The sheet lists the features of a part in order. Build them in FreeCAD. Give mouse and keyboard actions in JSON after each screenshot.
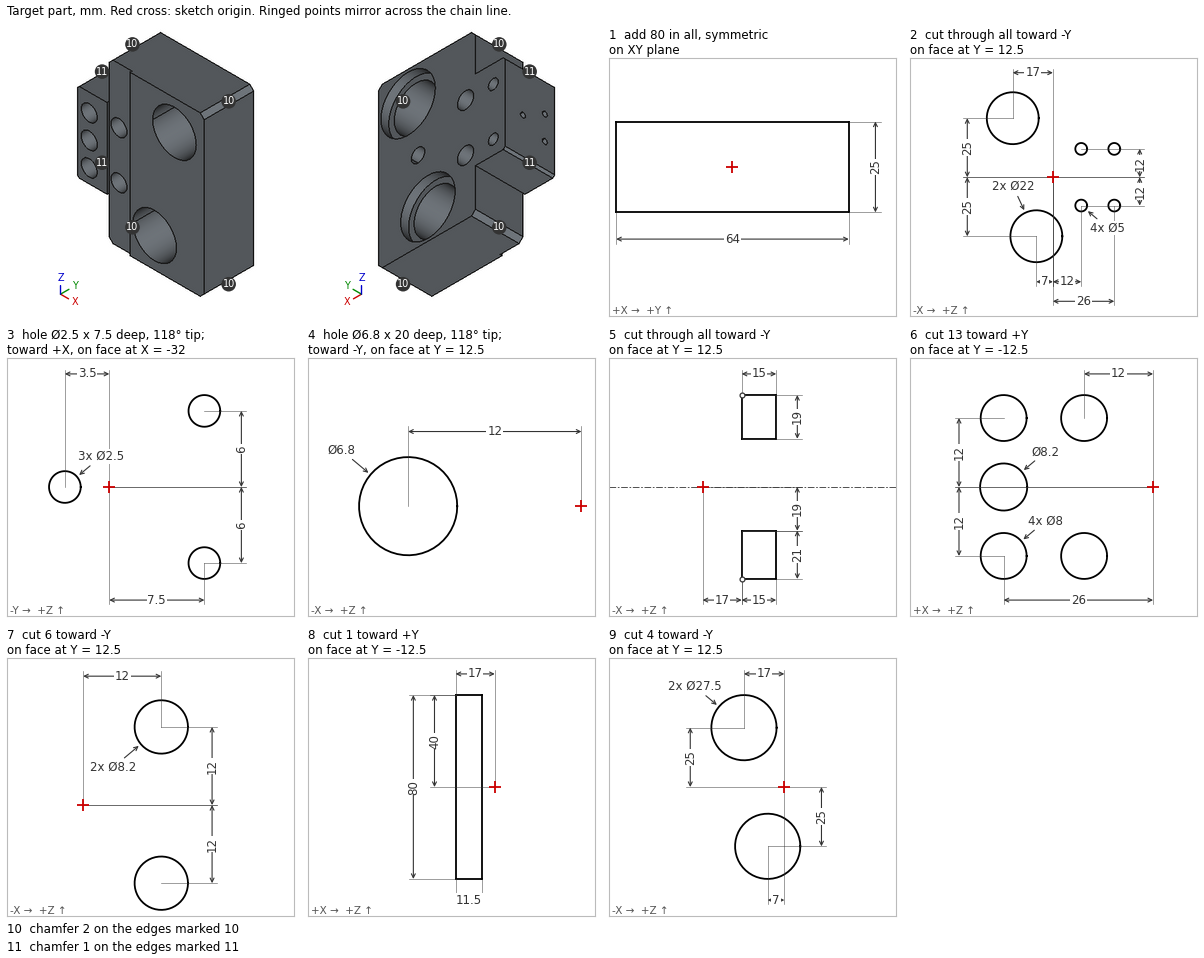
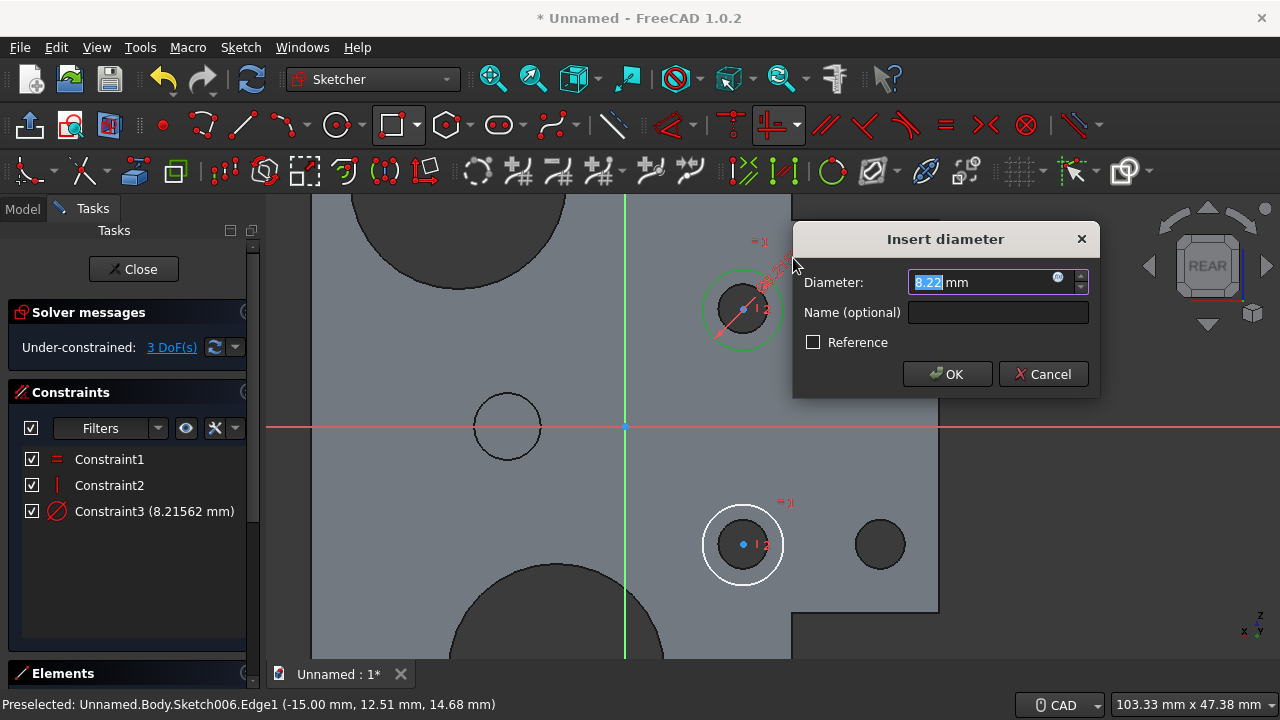
{"action": "type", "text": "8.2"}
{"action": "key", "text": "Return"}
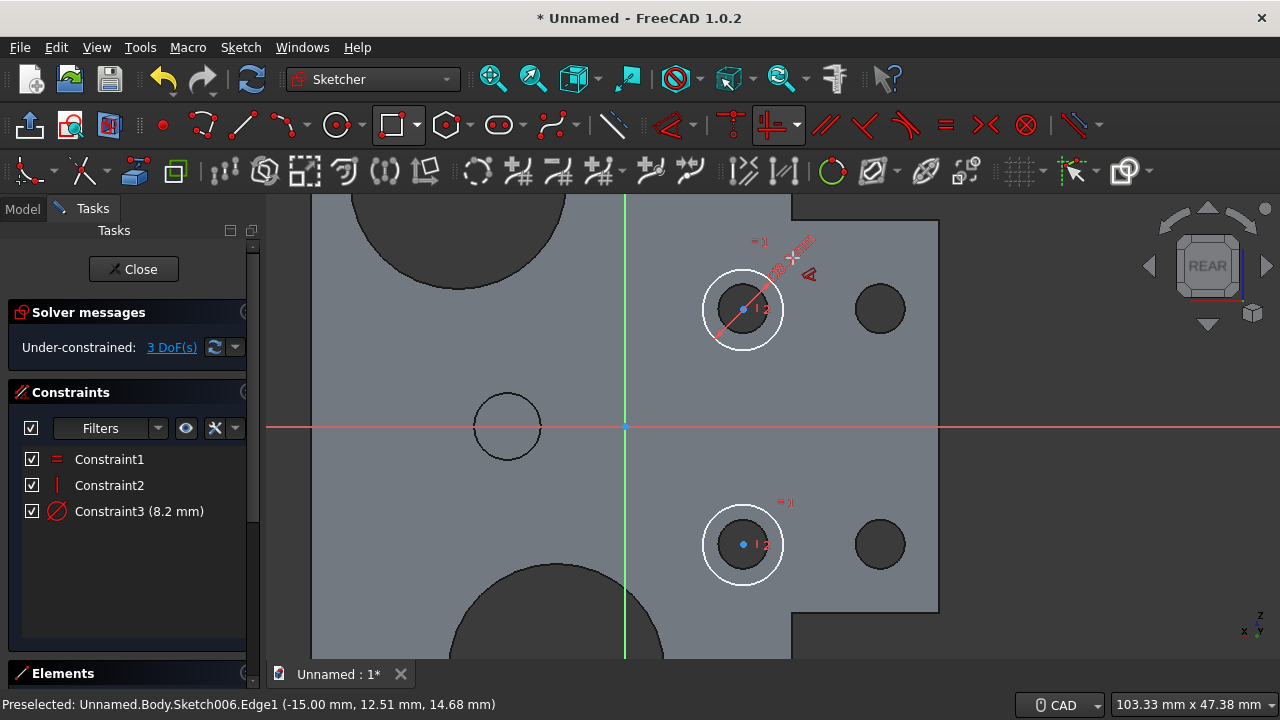
{"action": "left_click", "coordinate": [743, 310]}
{"action": "left_click", "coordinate": [684, 276]}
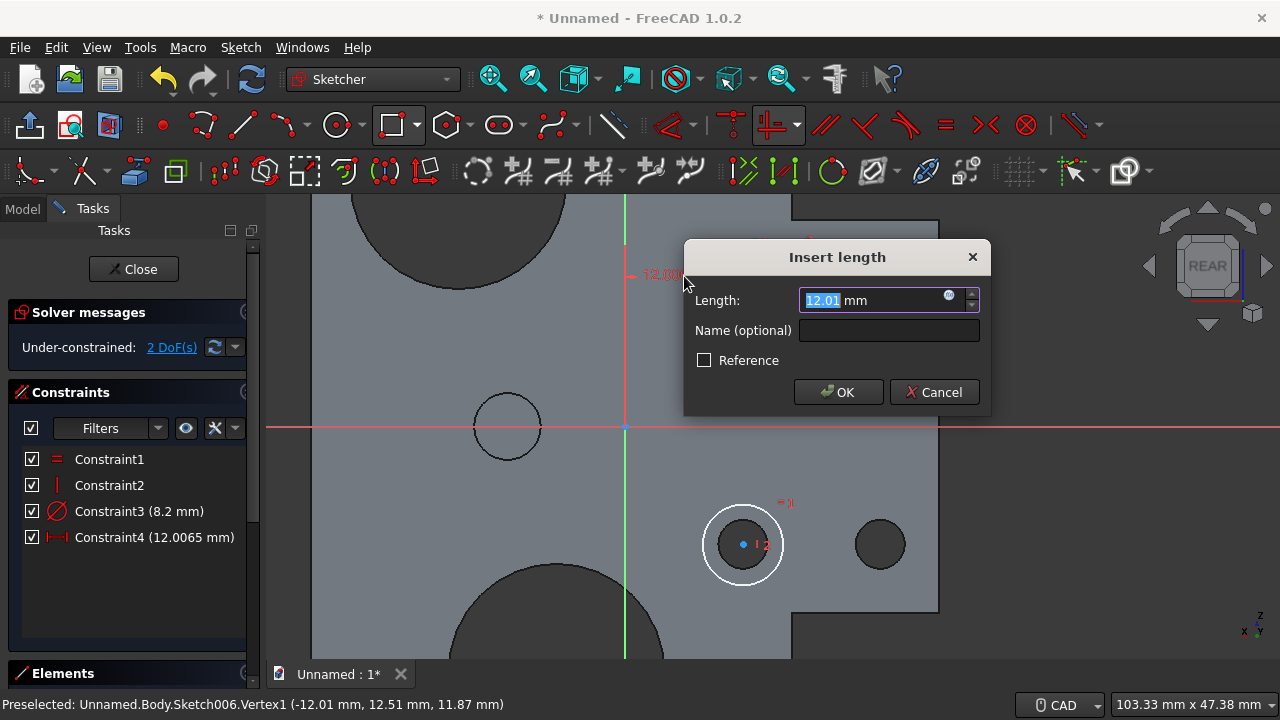
{"action": "type", "text": "12"}
{"action": "key", "text": "Return"}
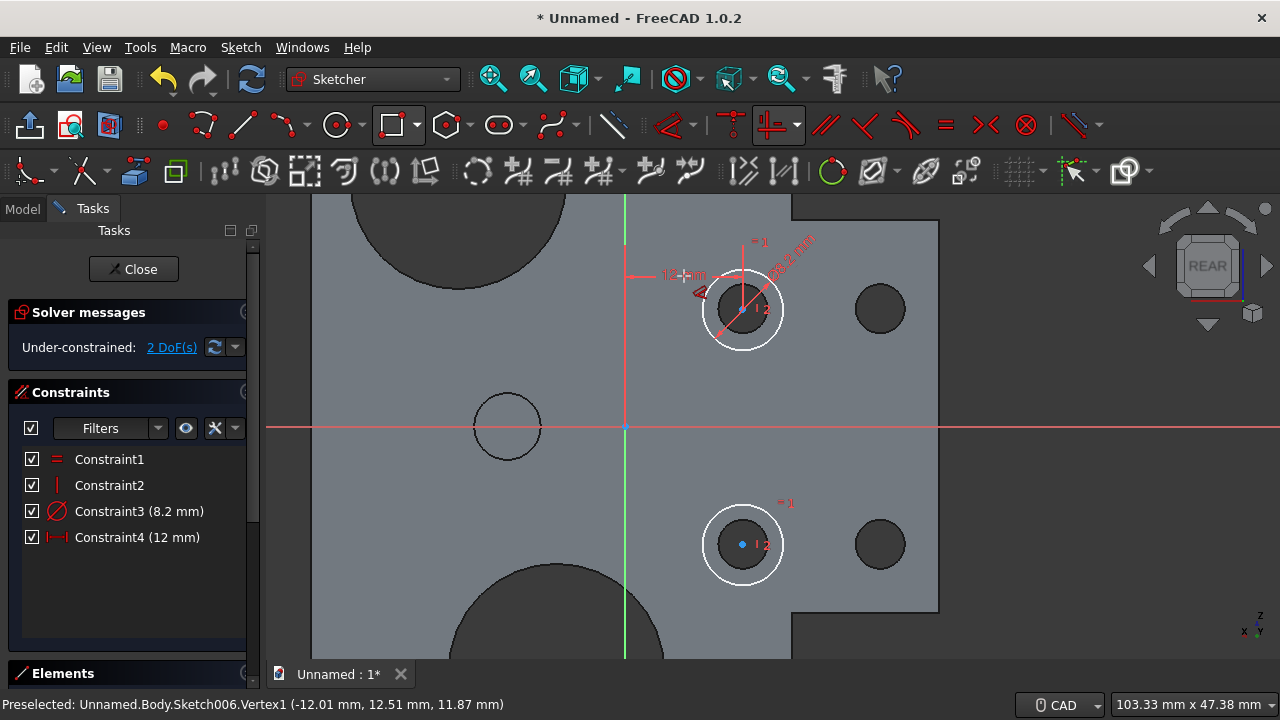
{"action": "left_click", "coordinate": [743, 310]}
{"action": "left_click", "coordinate": [591, 368]}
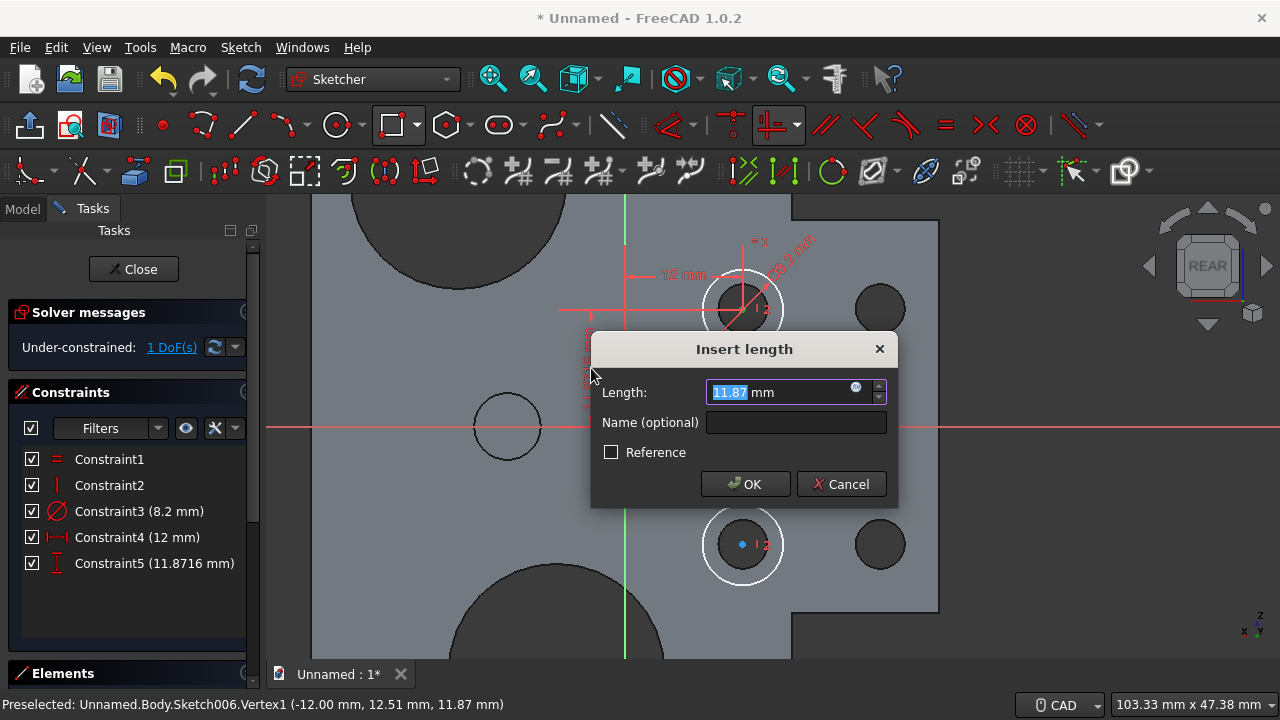
{"action": "type", "text": "12"}
{"action": "key", "text": "Return"}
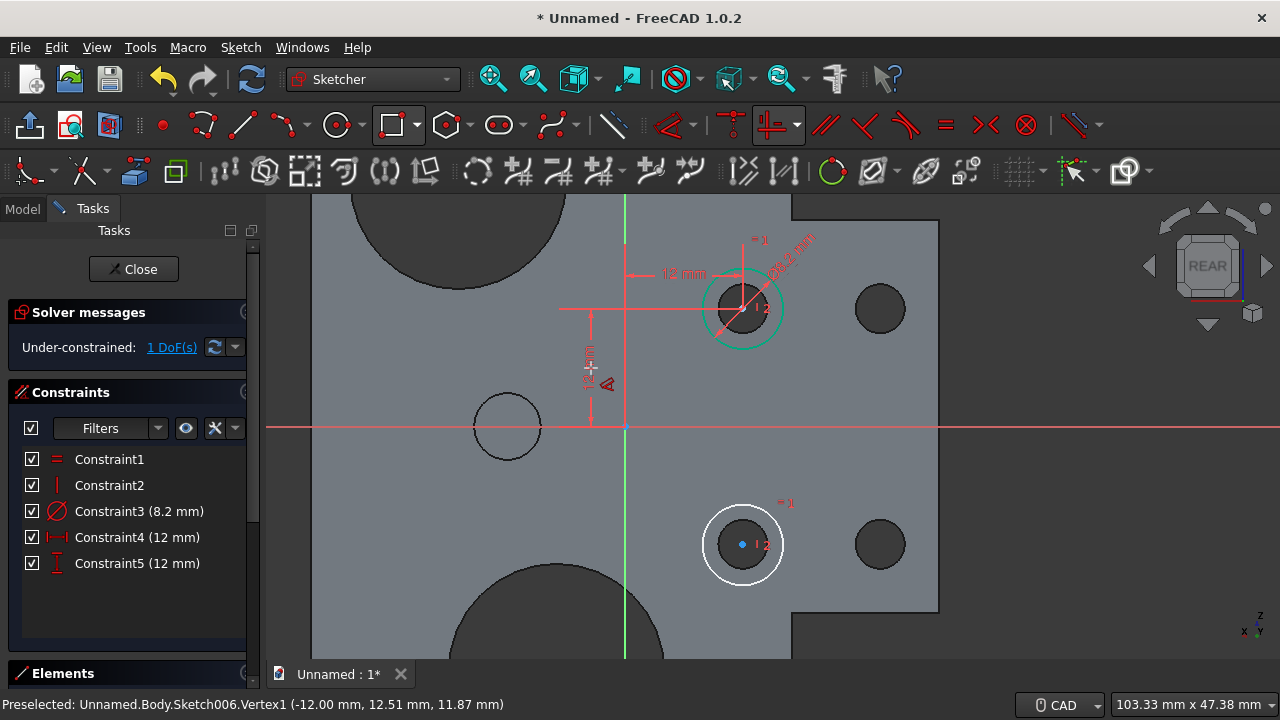
{"action": "left_click", "coordinate": [743, 545]}
{"action": "left_click", "coordinate": [591, 486]}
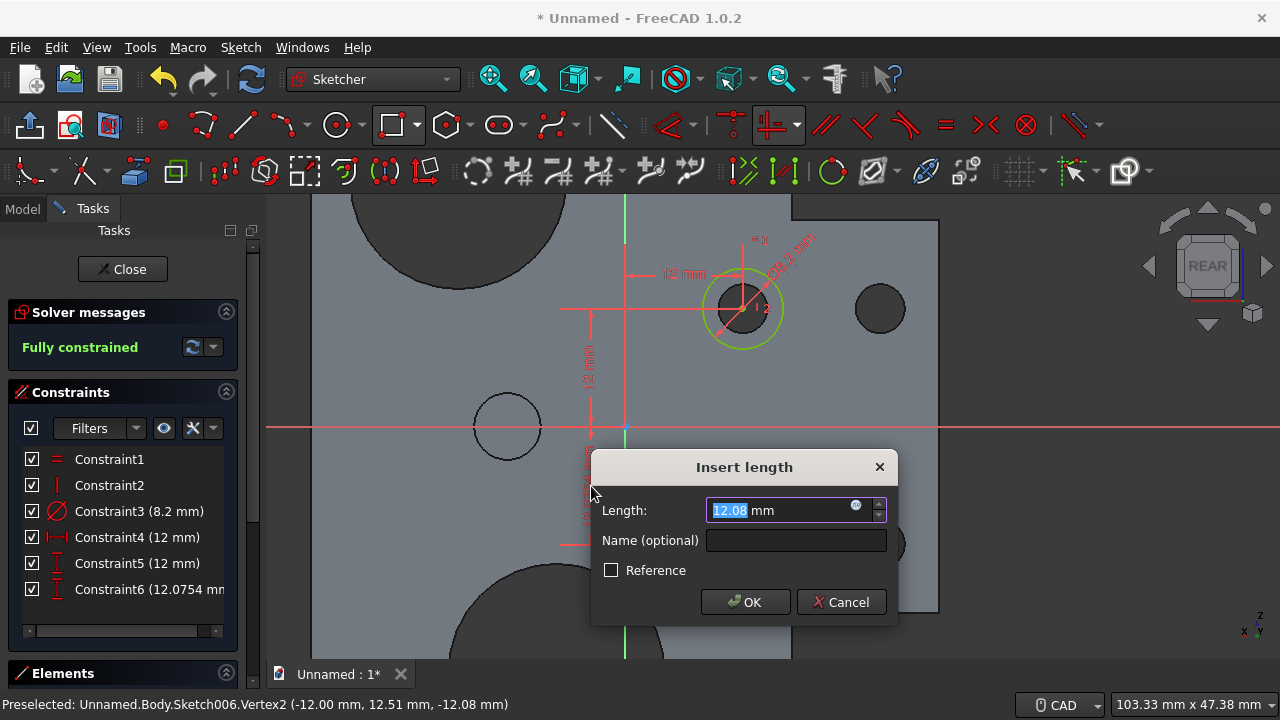
{"action": "type", "text": "12"}
{"action": "key", "text": "Return"}
{"action": "key", "text": "Escape"}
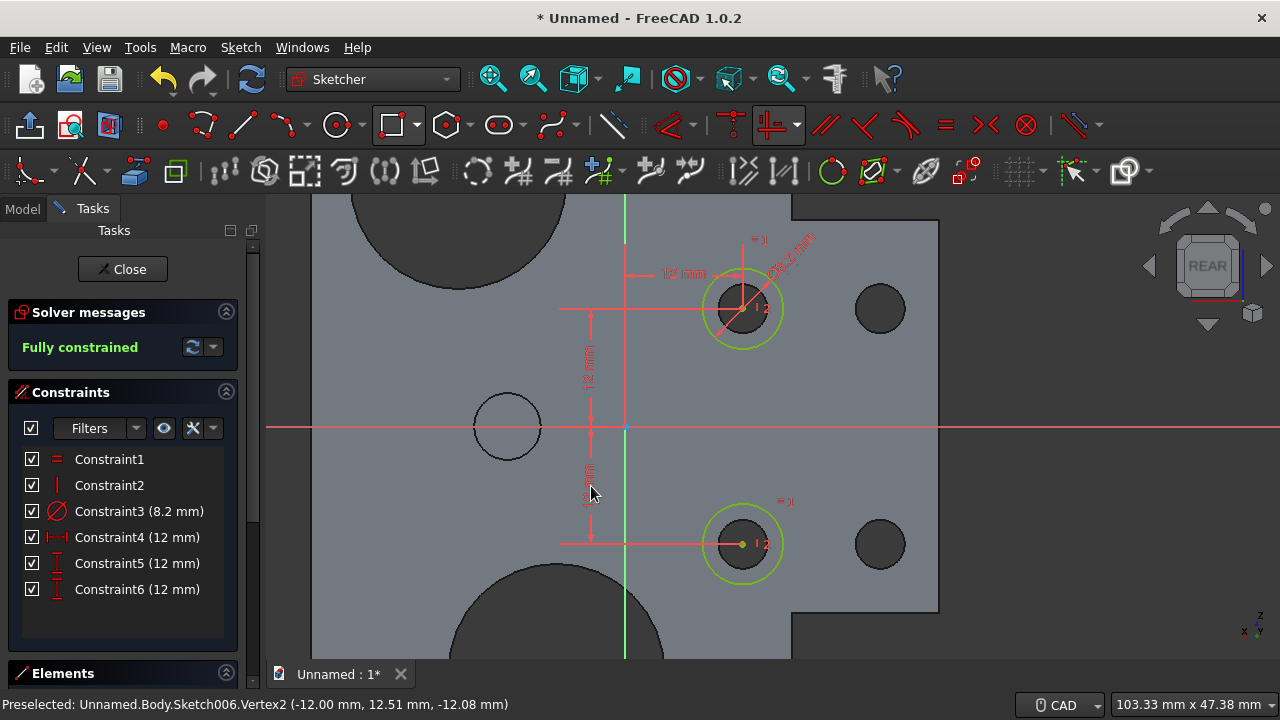
{"action": "left_click", "coordinate": [123, 269]}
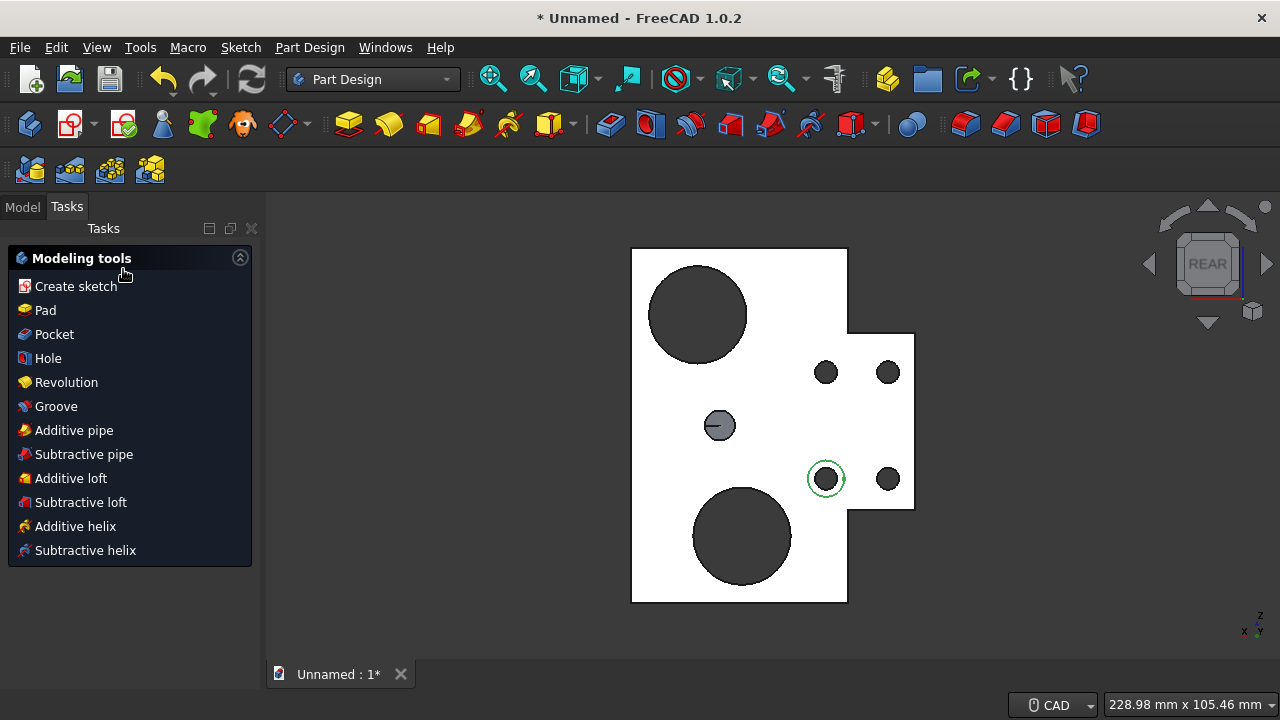
{"action": "left_click", "coordinate": [612, 124]}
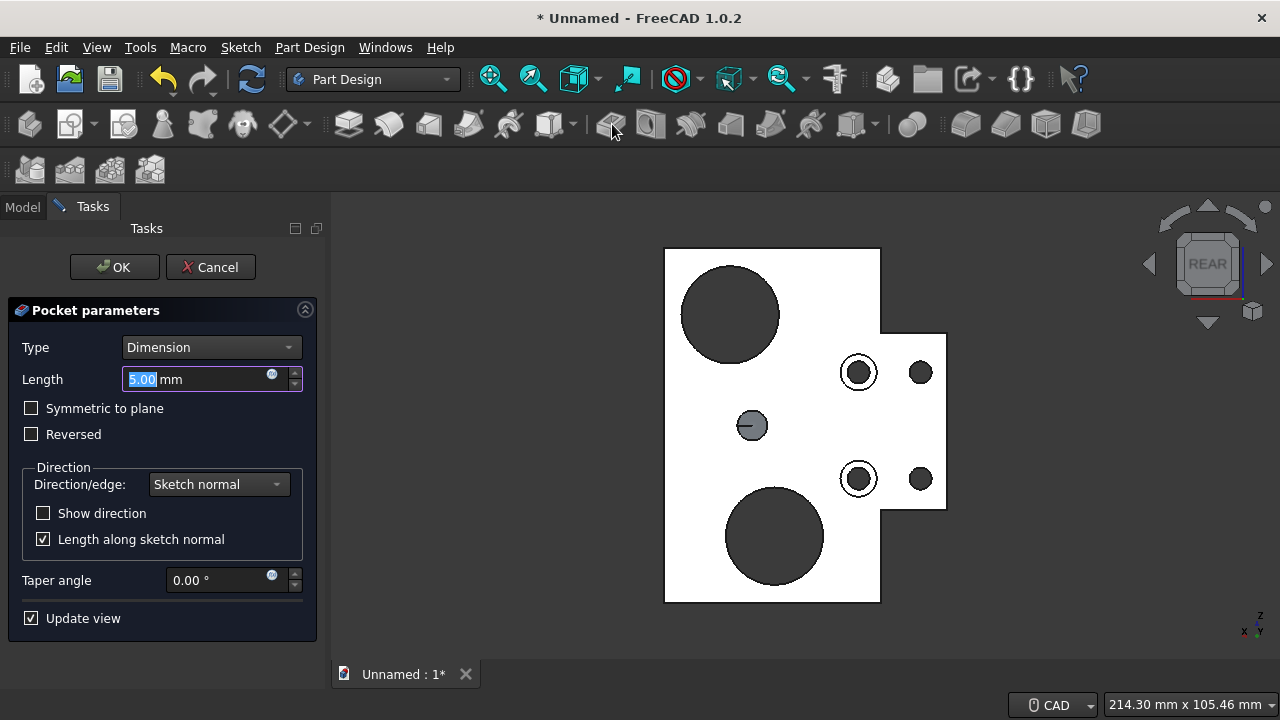
{"action": "type", "text": "6"}
{"action": "key", "text": "Tab"}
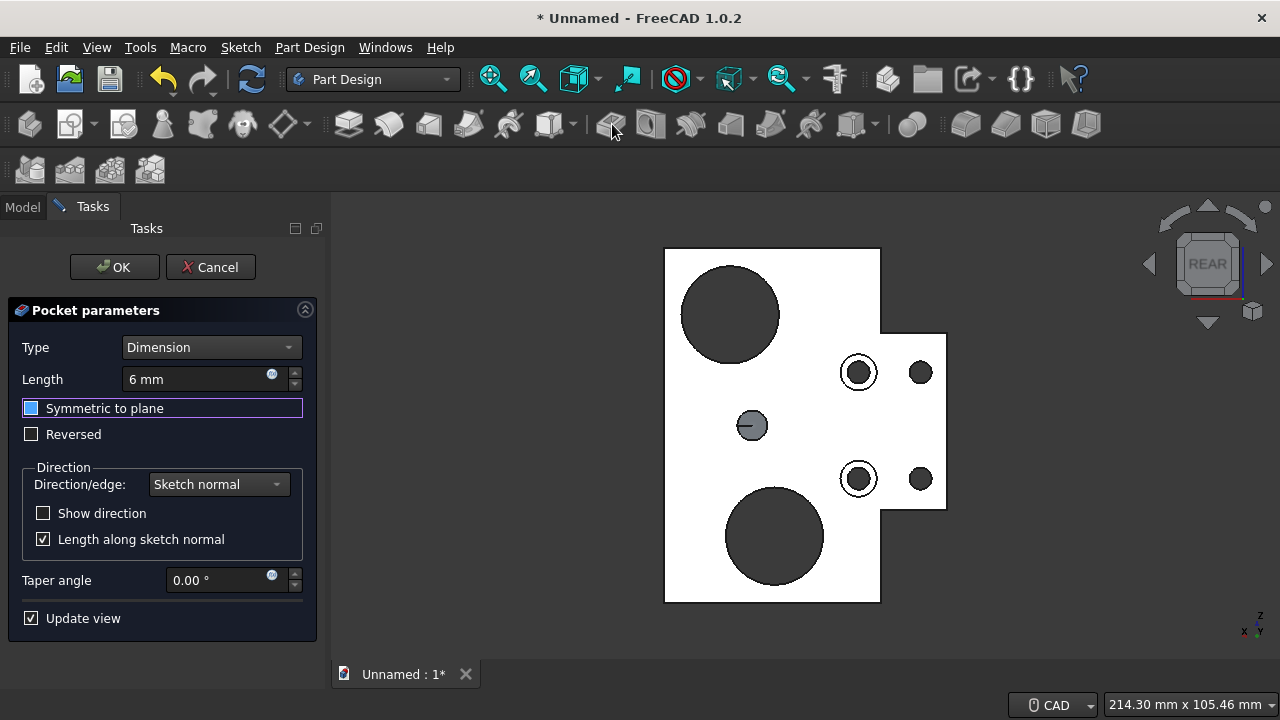
{"action": "left_click", "coordinate": [115, 267]}